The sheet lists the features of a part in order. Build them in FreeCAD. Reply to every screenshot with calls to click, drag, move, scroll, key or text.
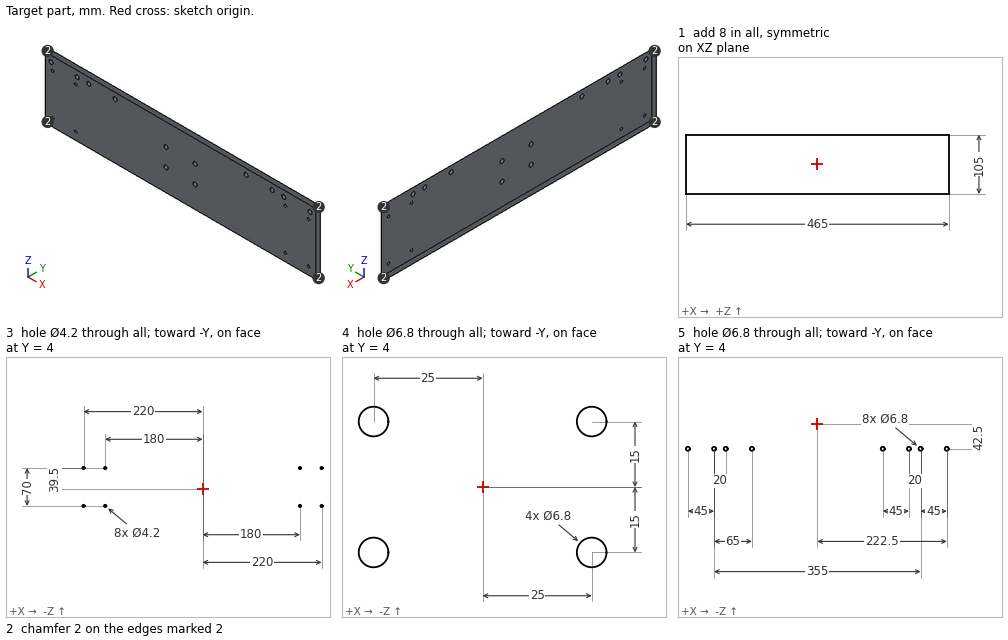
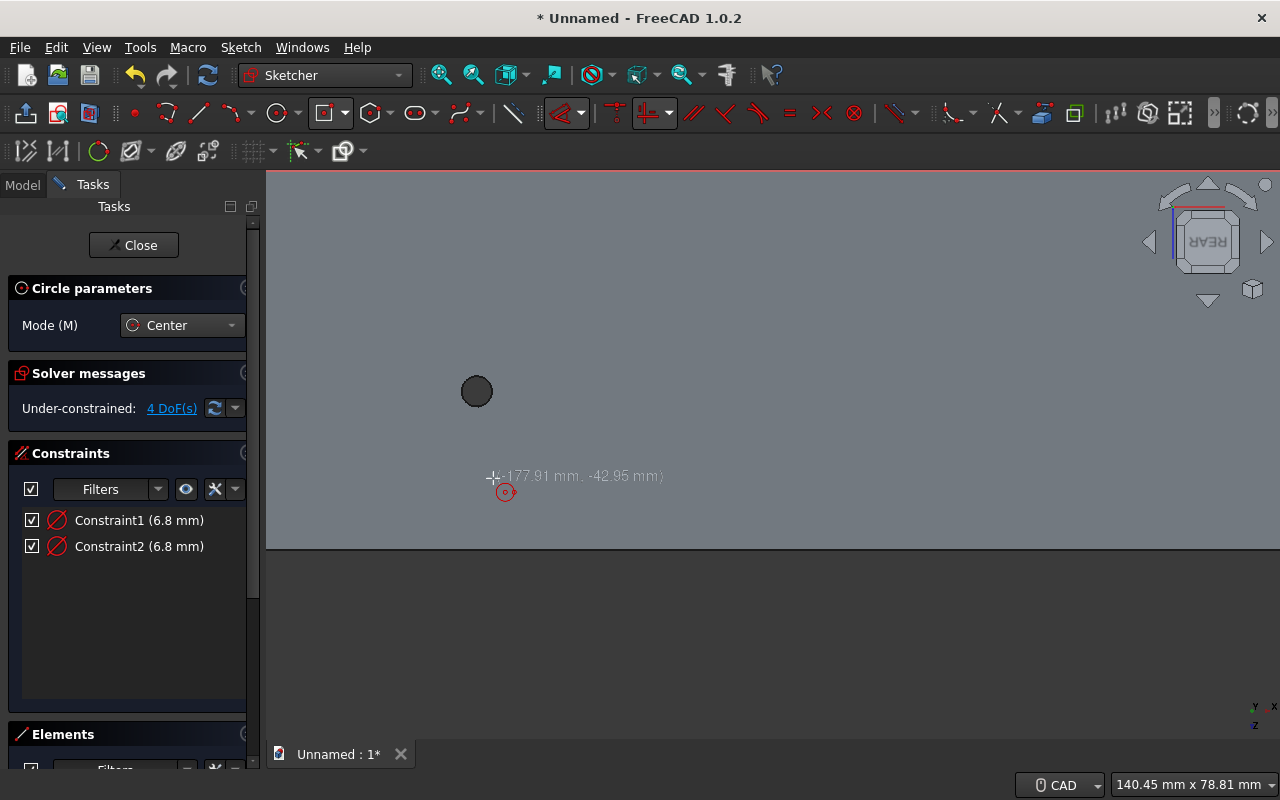
scroll(492, 478, down, 9)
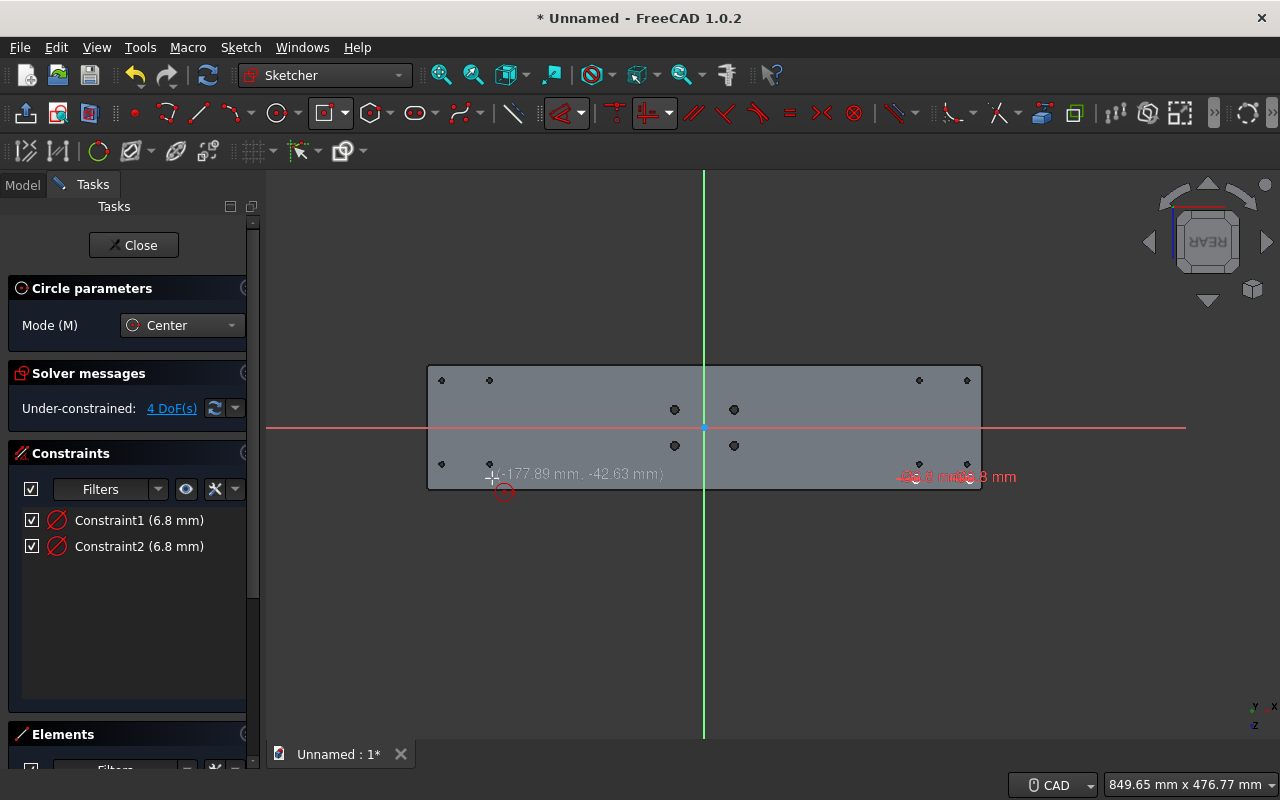
click(493, 478)
move(496, 476)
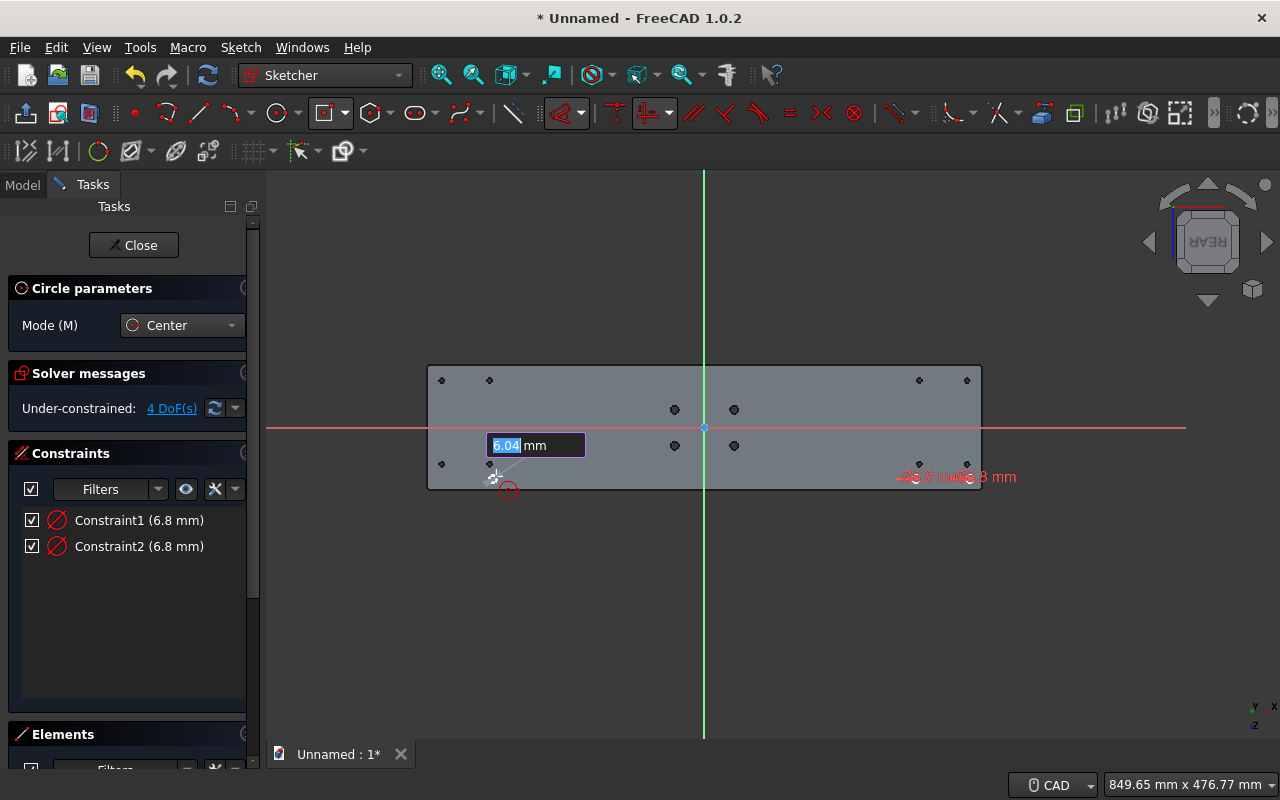
text(6.8)
key(Return)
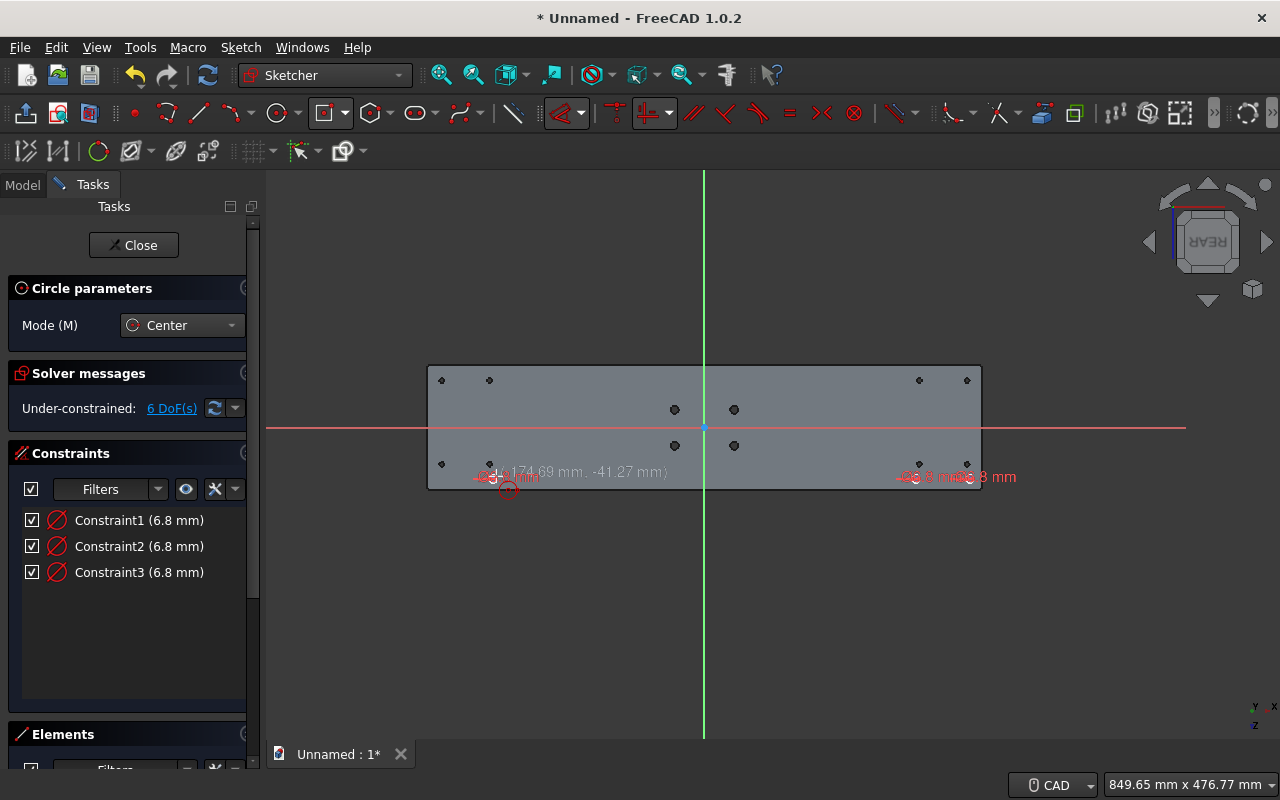
scroll(439, 478, up, 9)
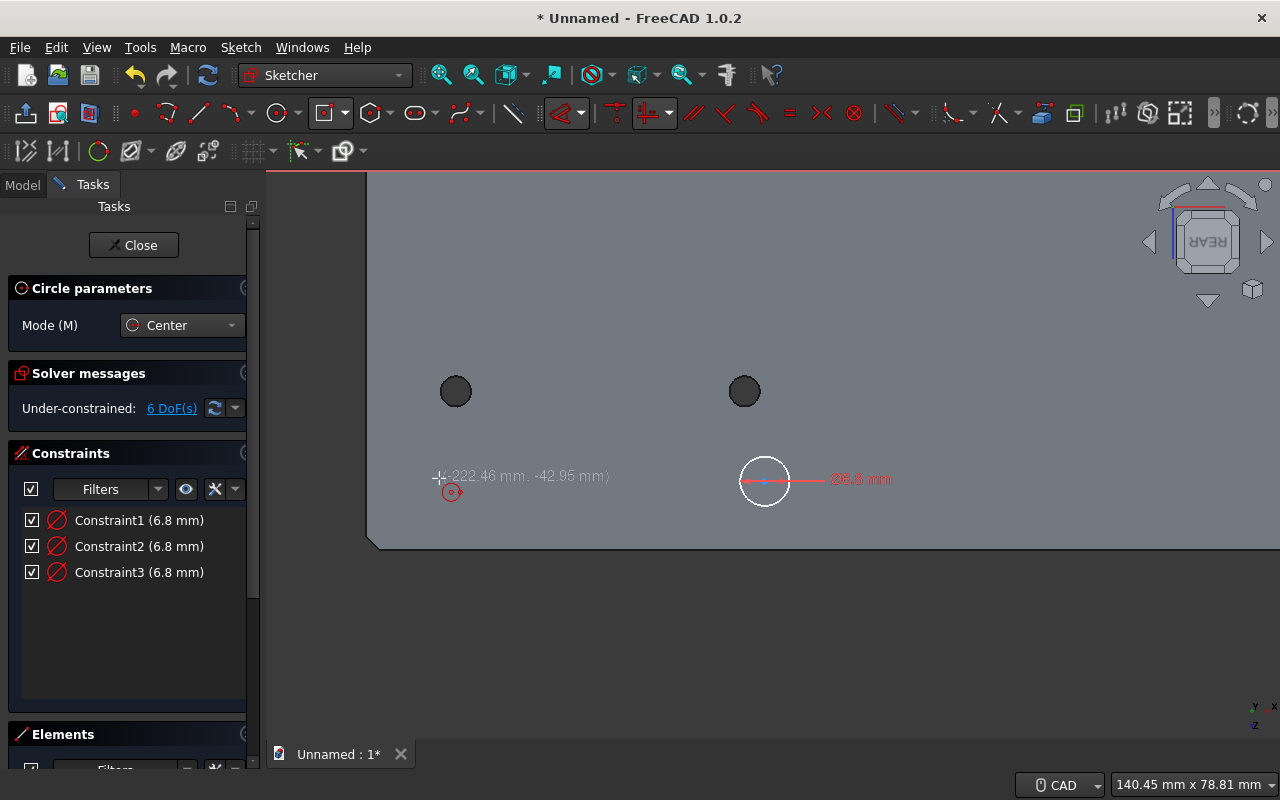
scroll(439, 478, down, 9)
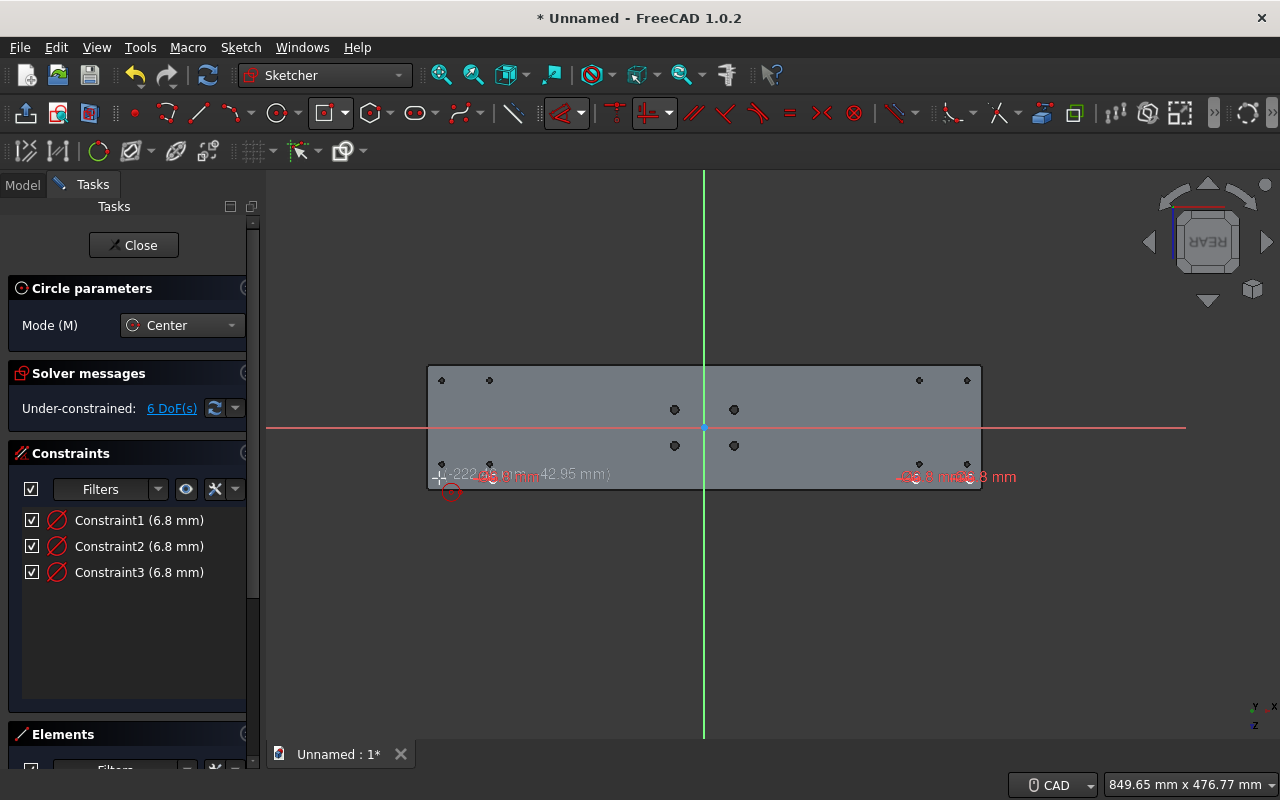
click(439, 478)
move(442, 476)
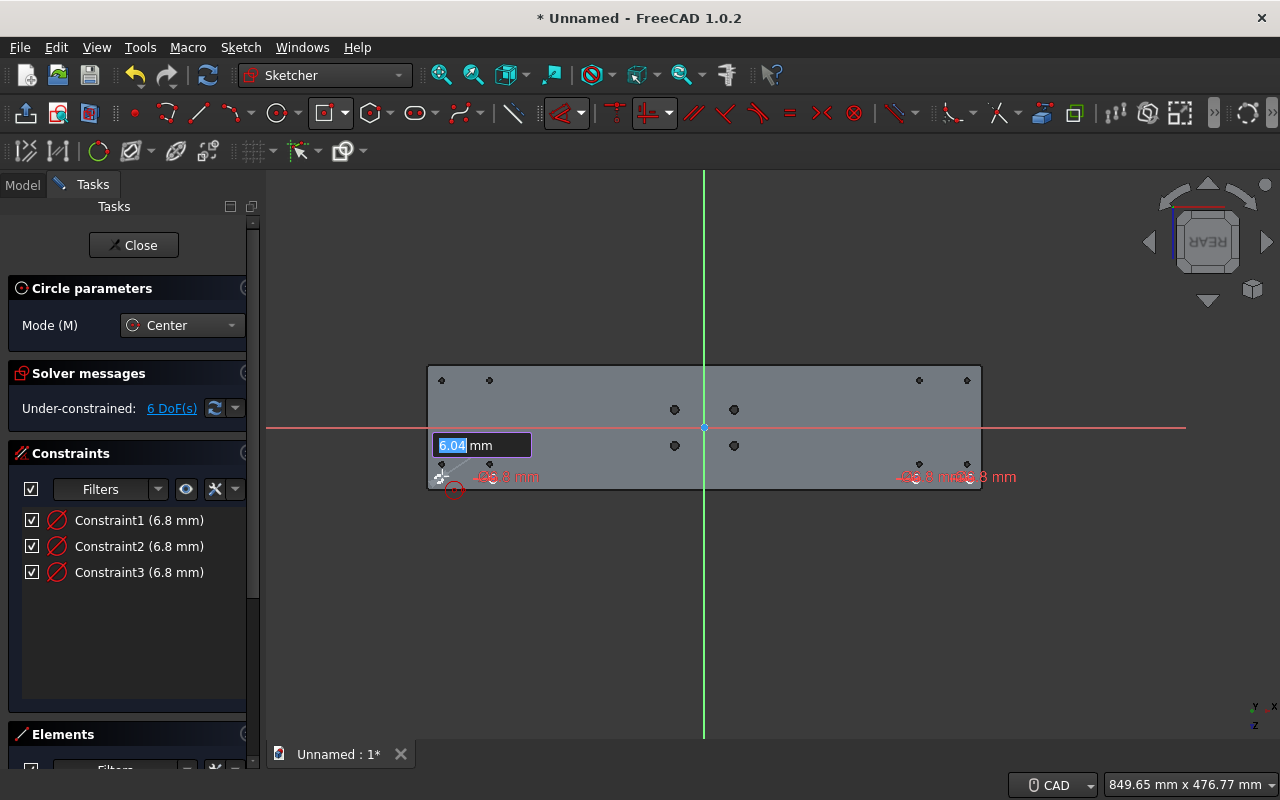
text(6.8)
key(Return)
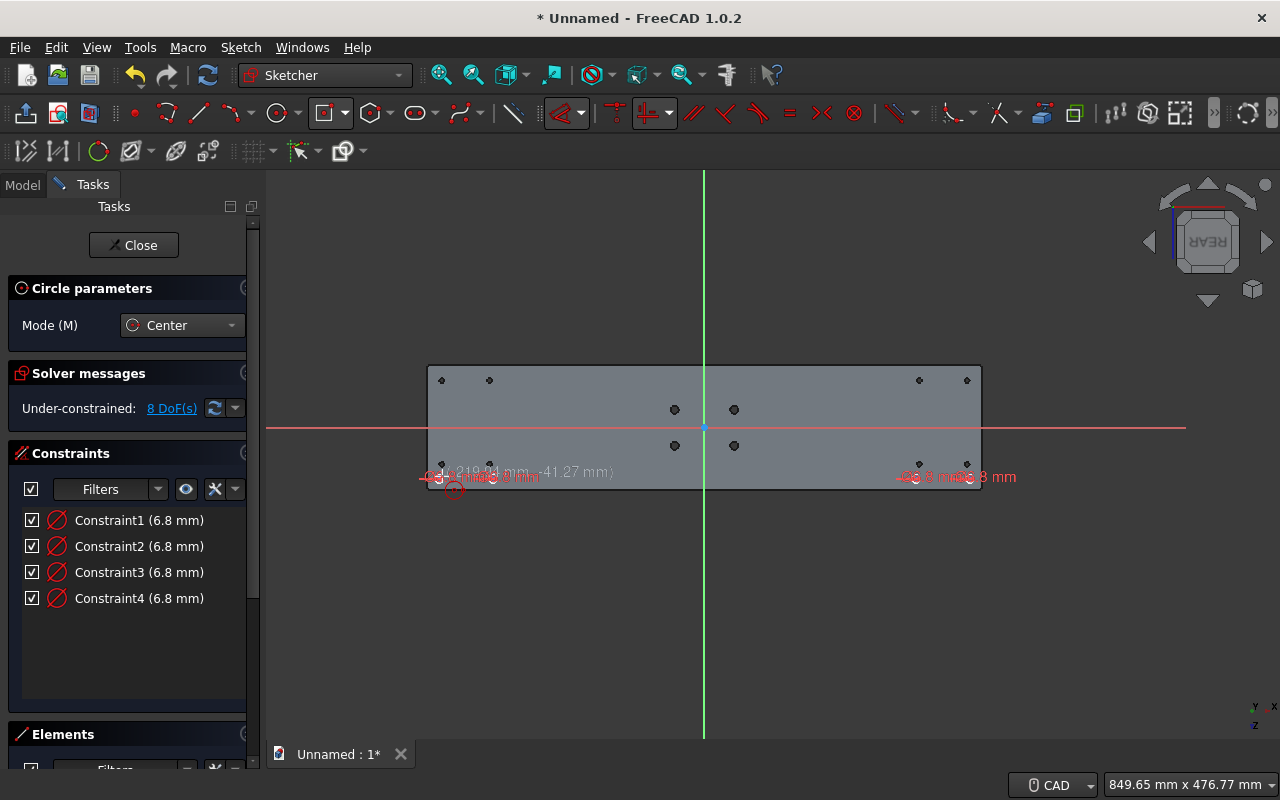
scroll(892, 478, up, 9)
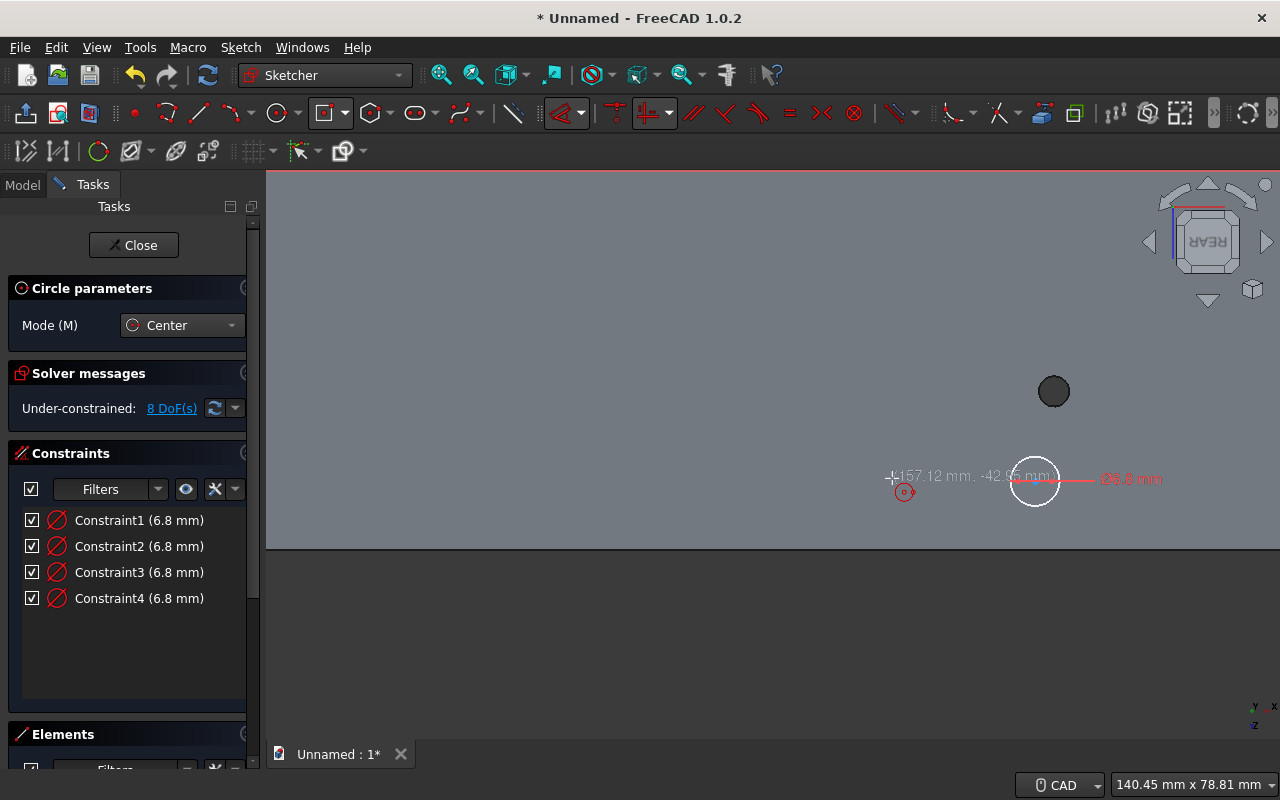
scroll(893, 478, down, 9)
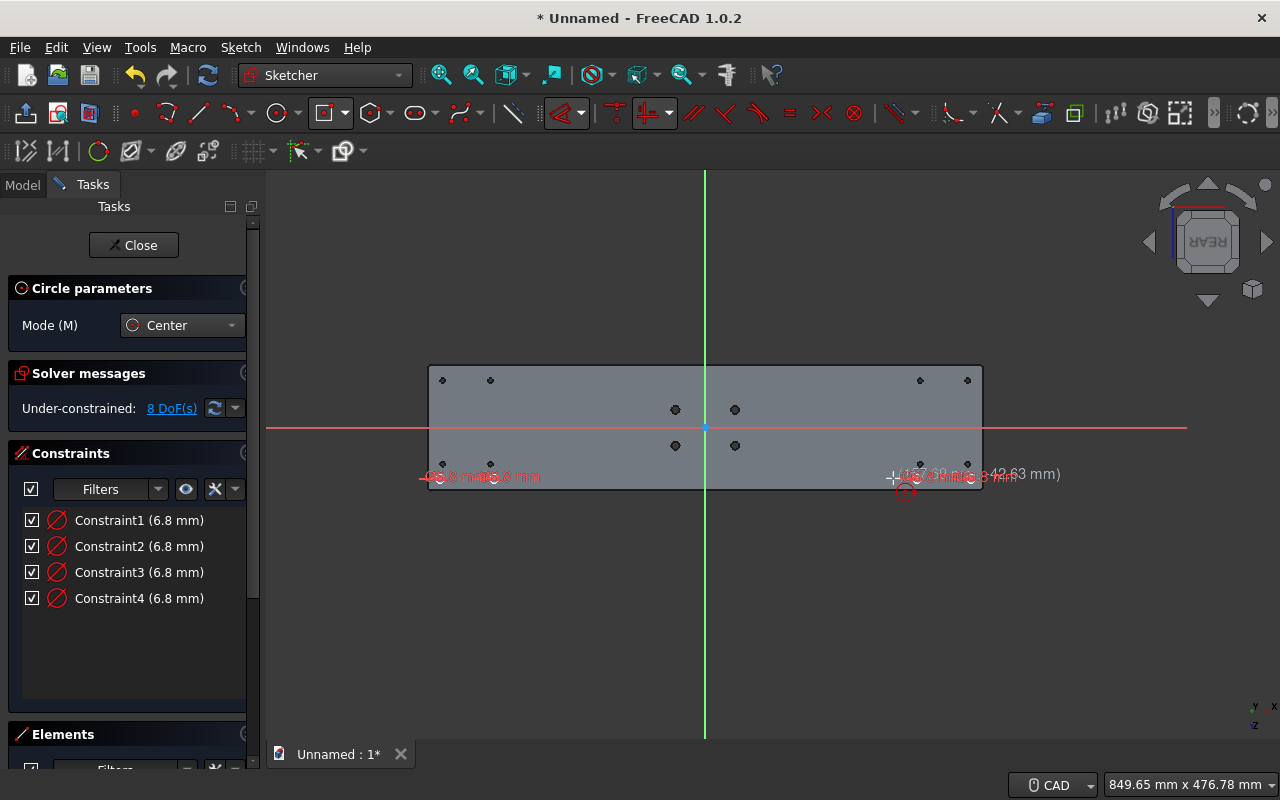
click(893, 478)
move(896, 476)